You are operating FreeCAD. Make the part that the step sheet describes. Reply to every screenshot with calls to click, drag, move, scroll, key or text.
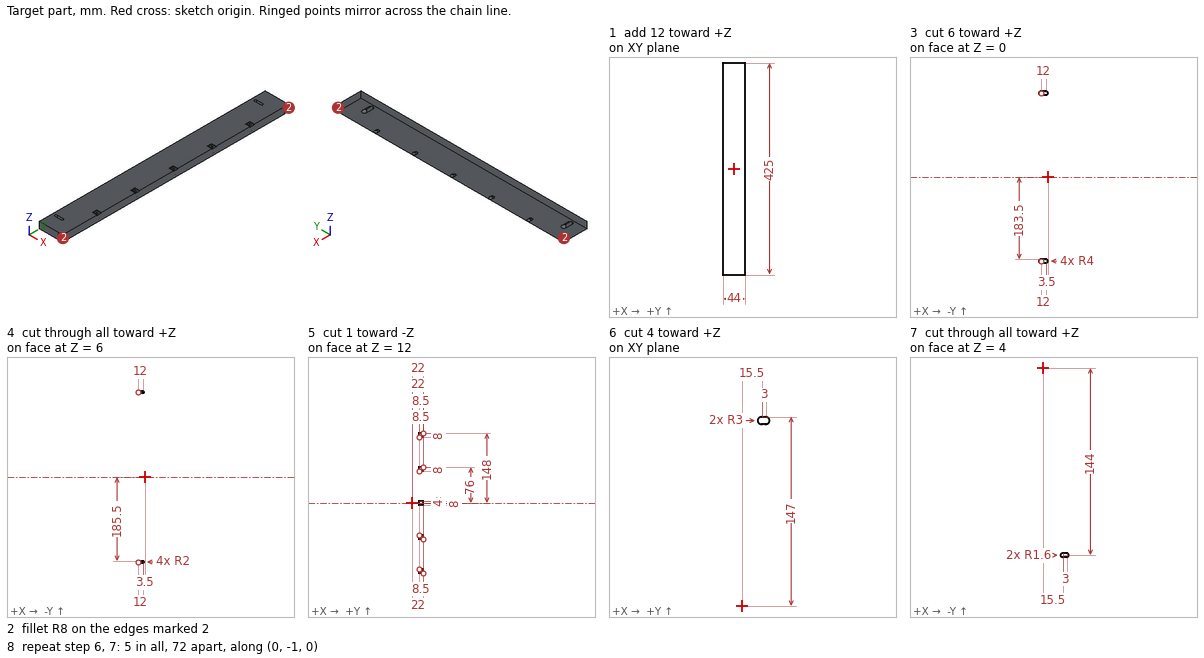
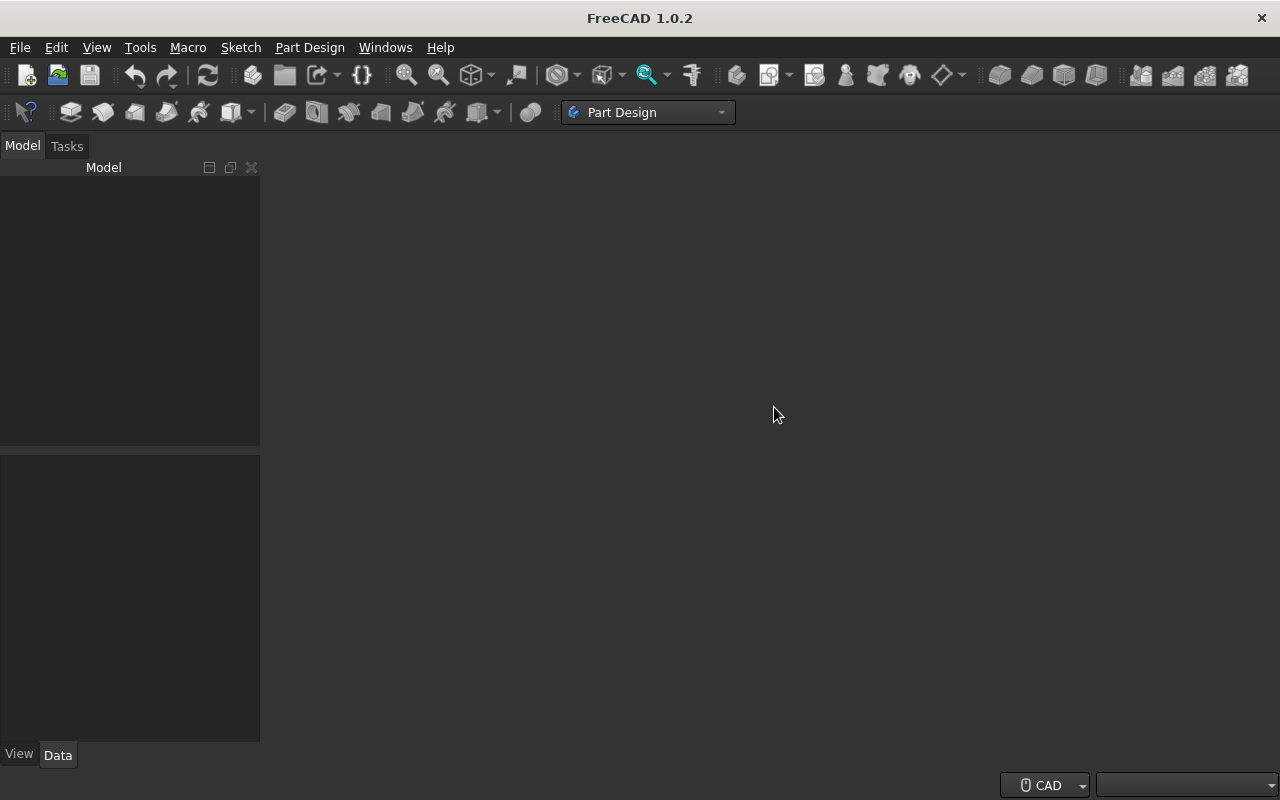
click(26, 76)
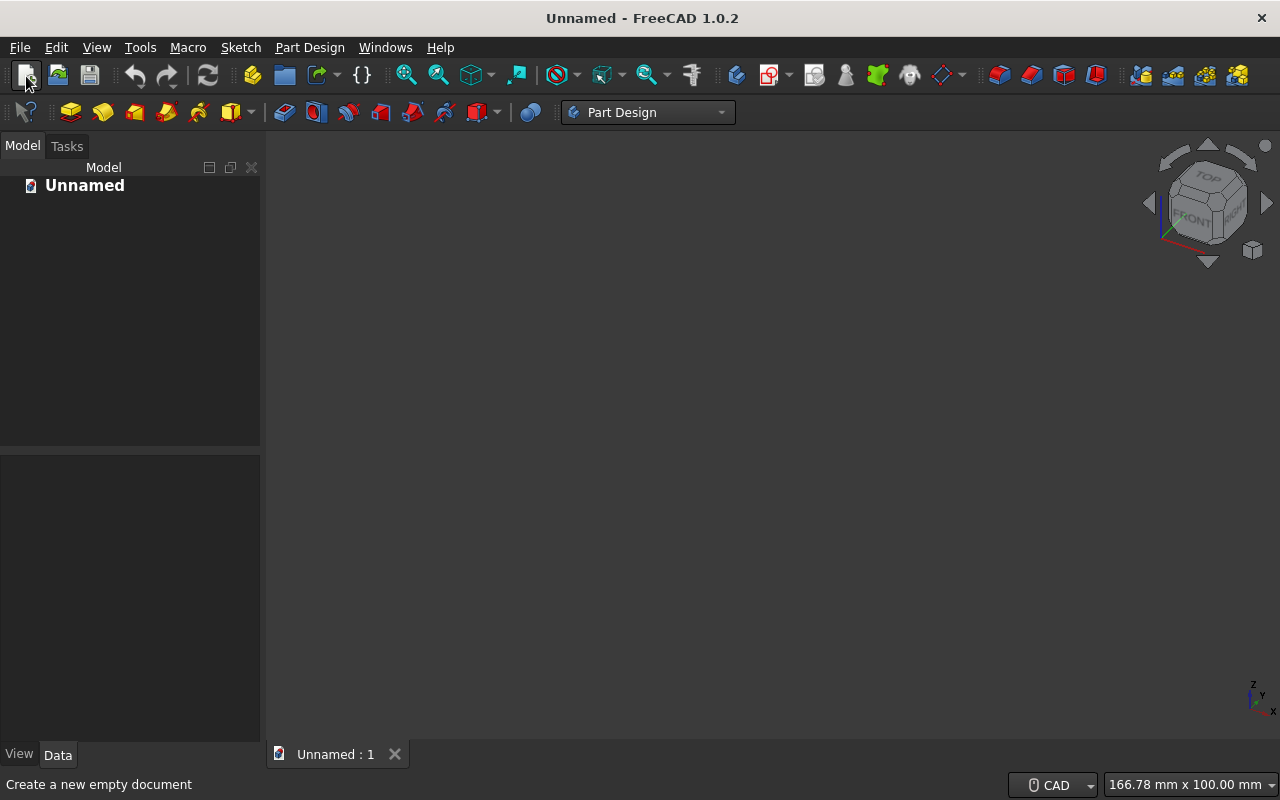
click(770, 76)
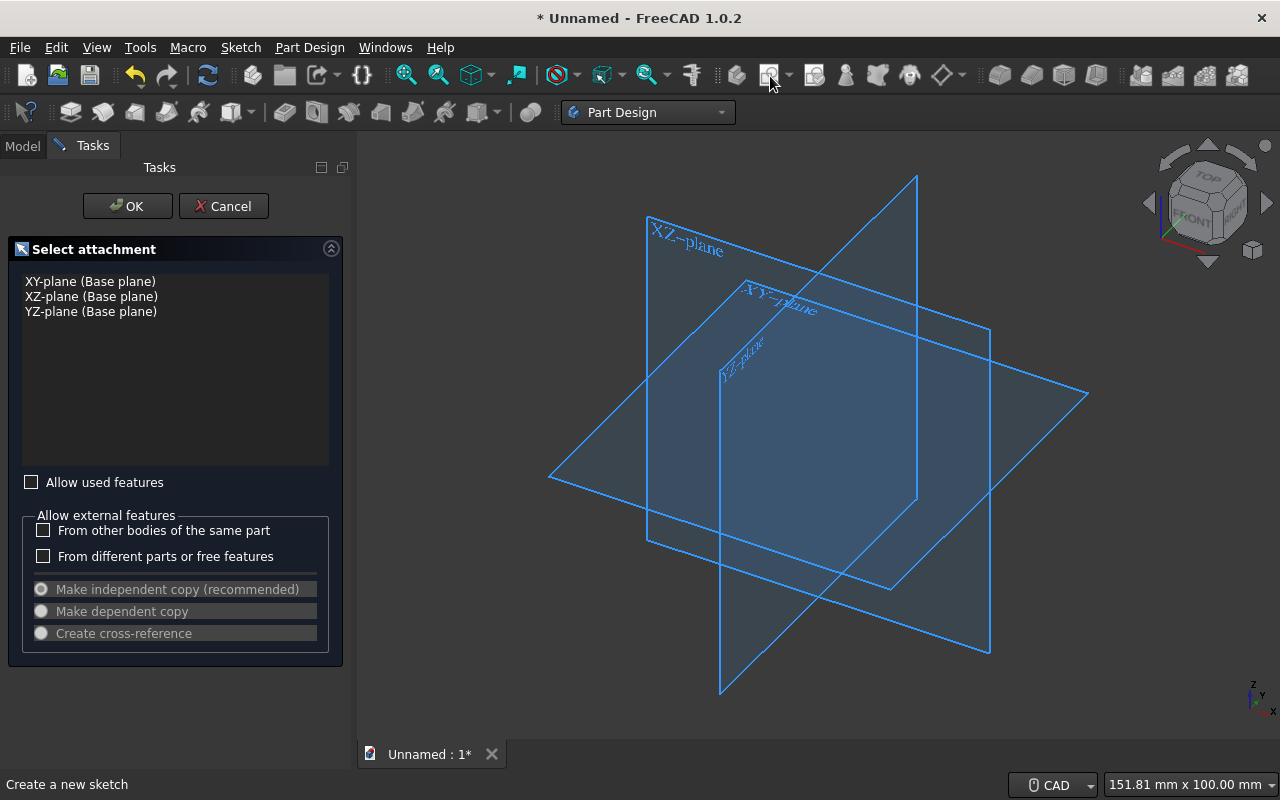
click(82, 282)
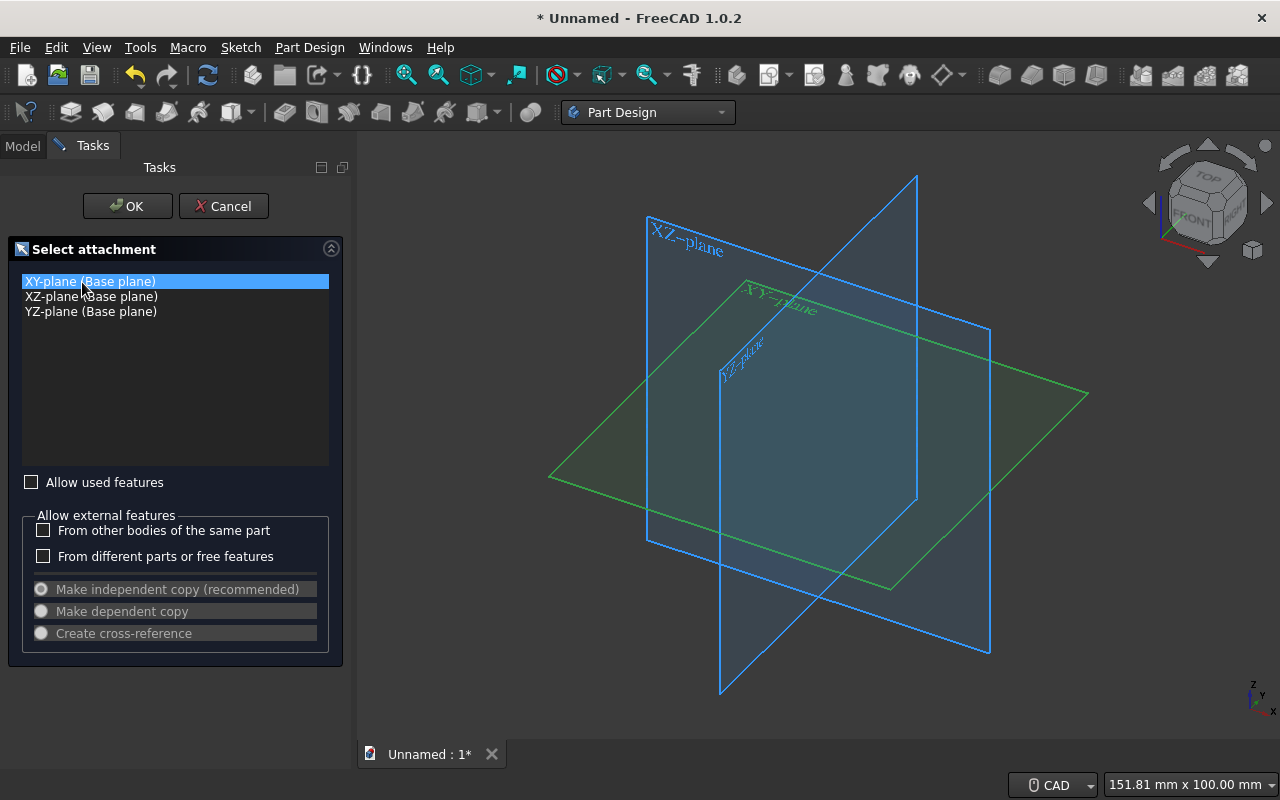
click(128, 206)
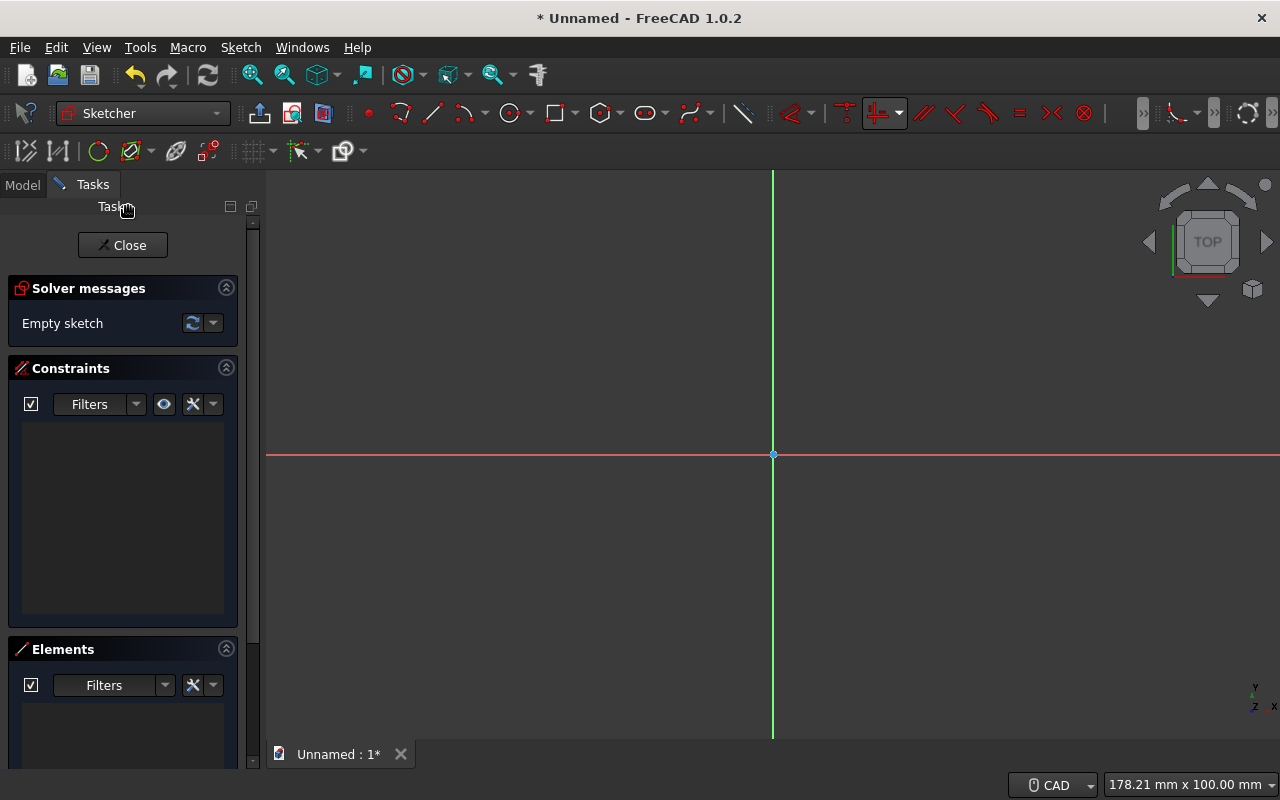
scroll(691, 454, down, 9)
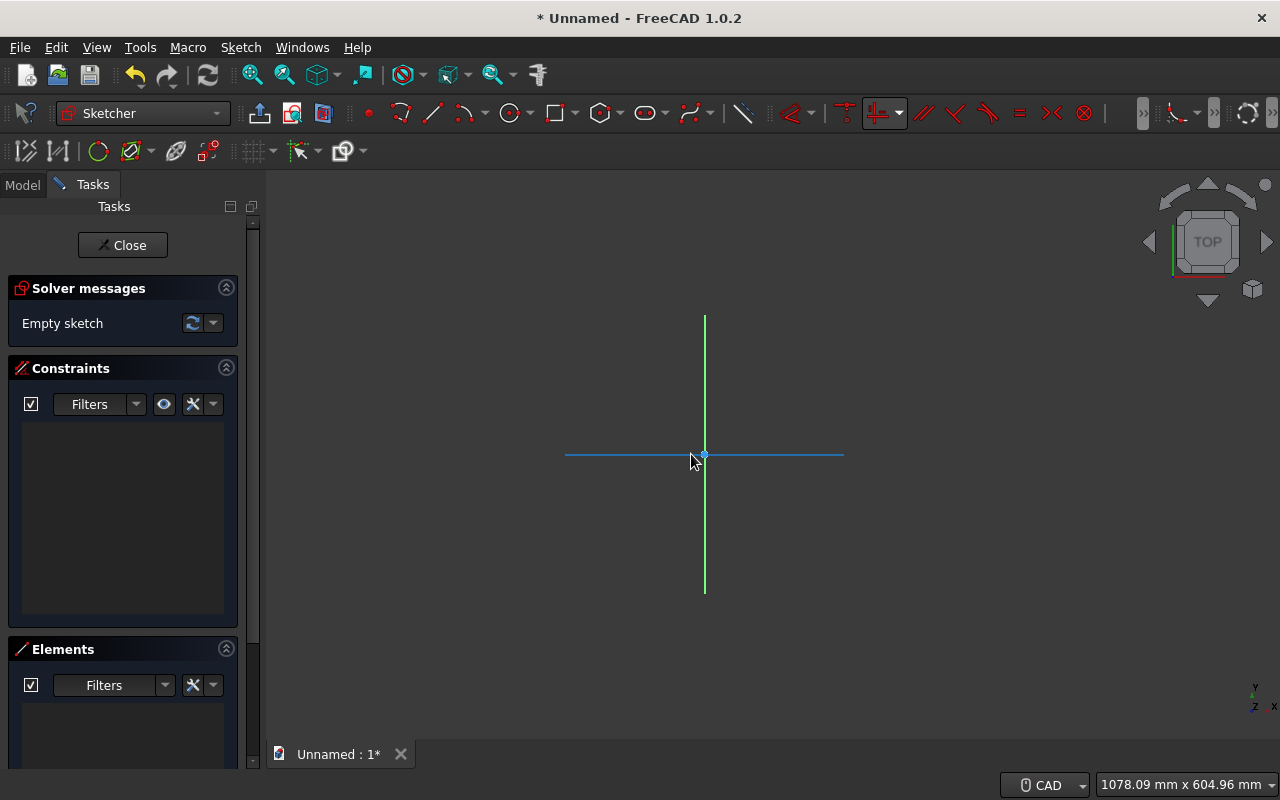
click(578, 114)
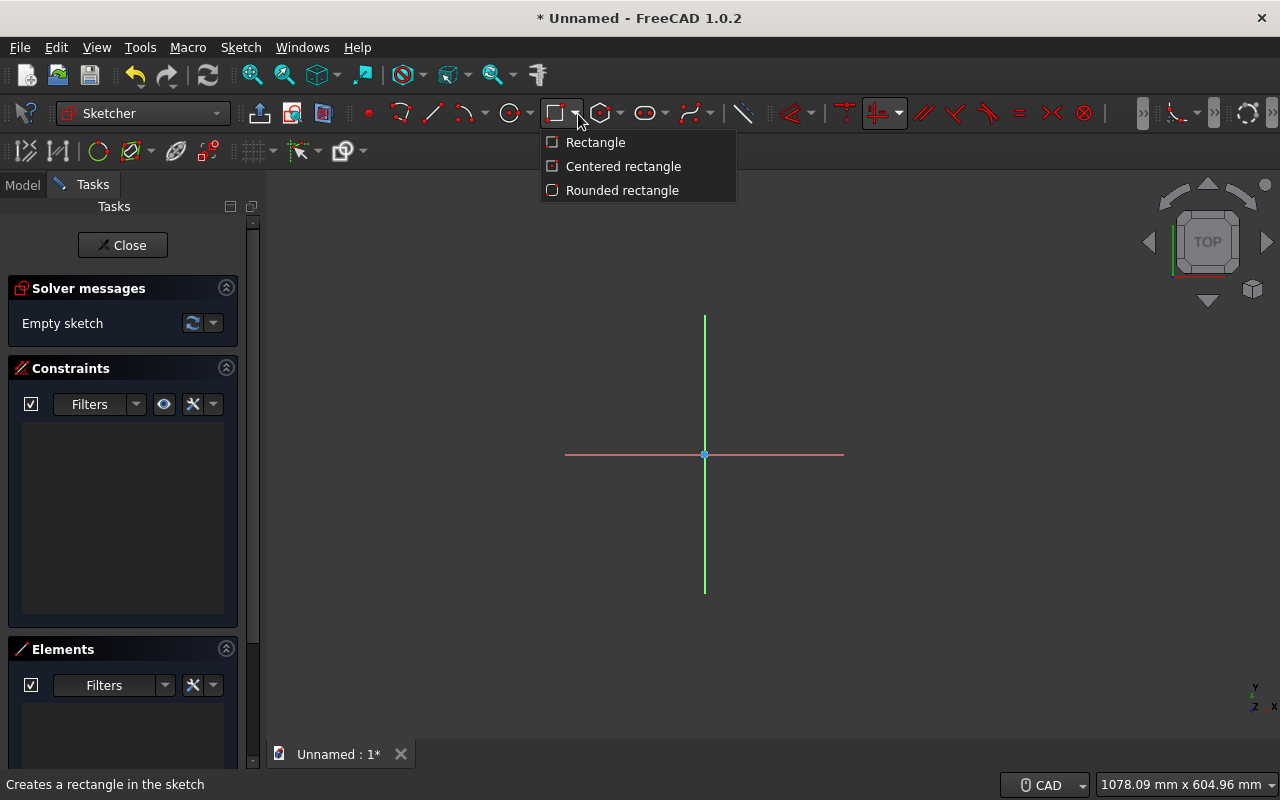
click(638, 166)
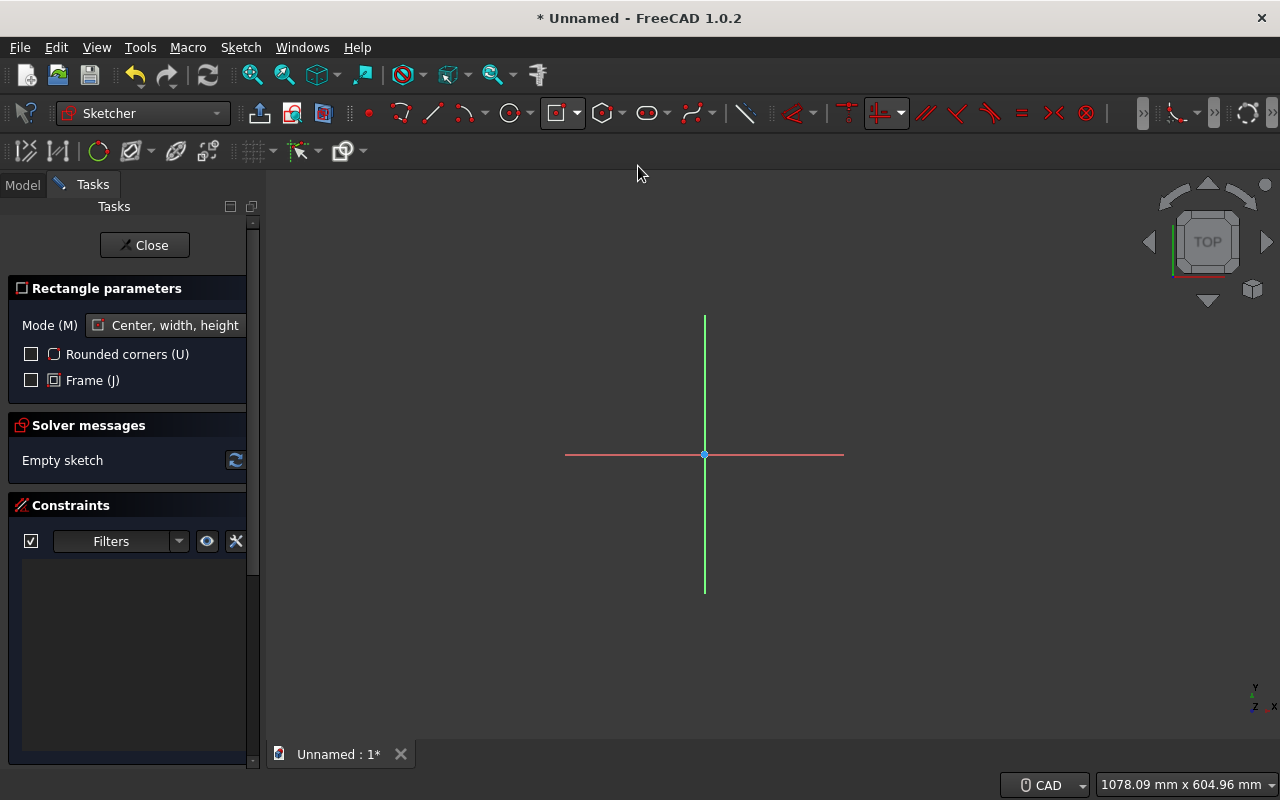
click(705, 454)
click(726, 255)
key(Escape)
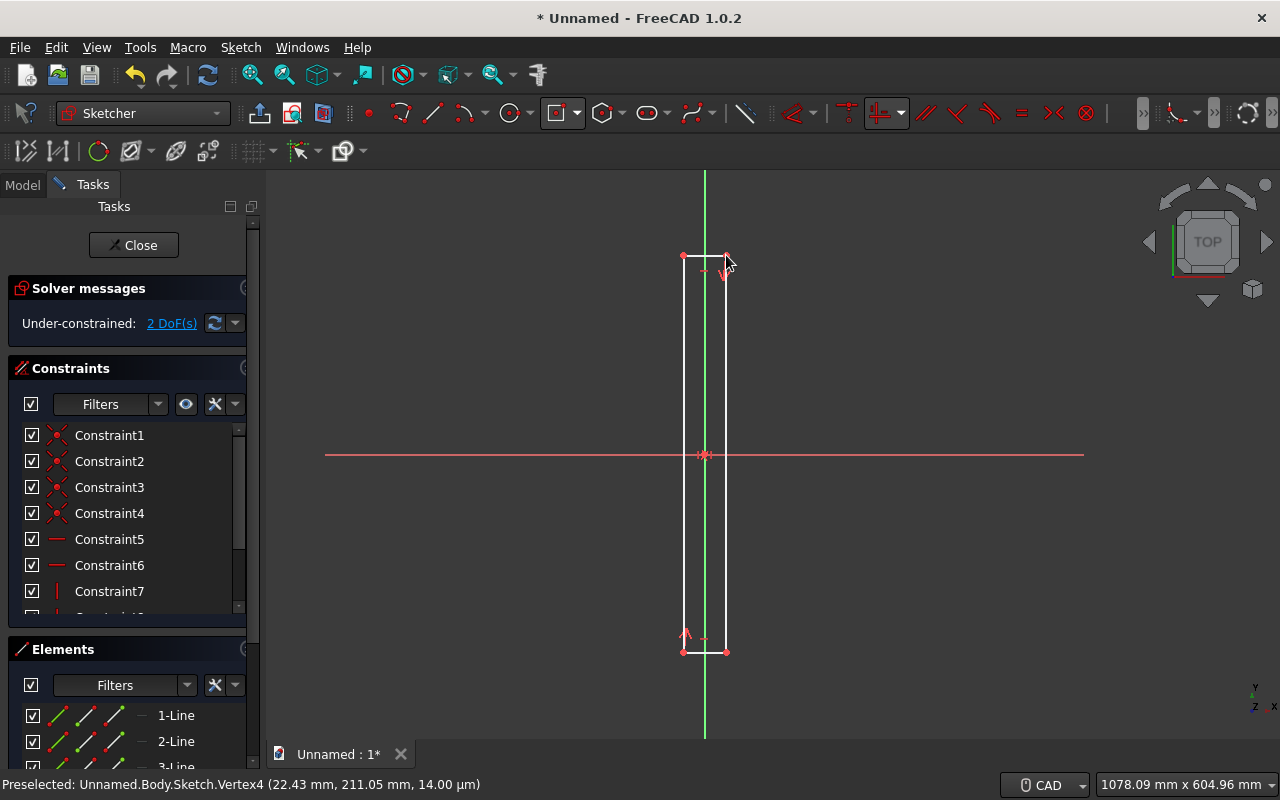
click(792, 114)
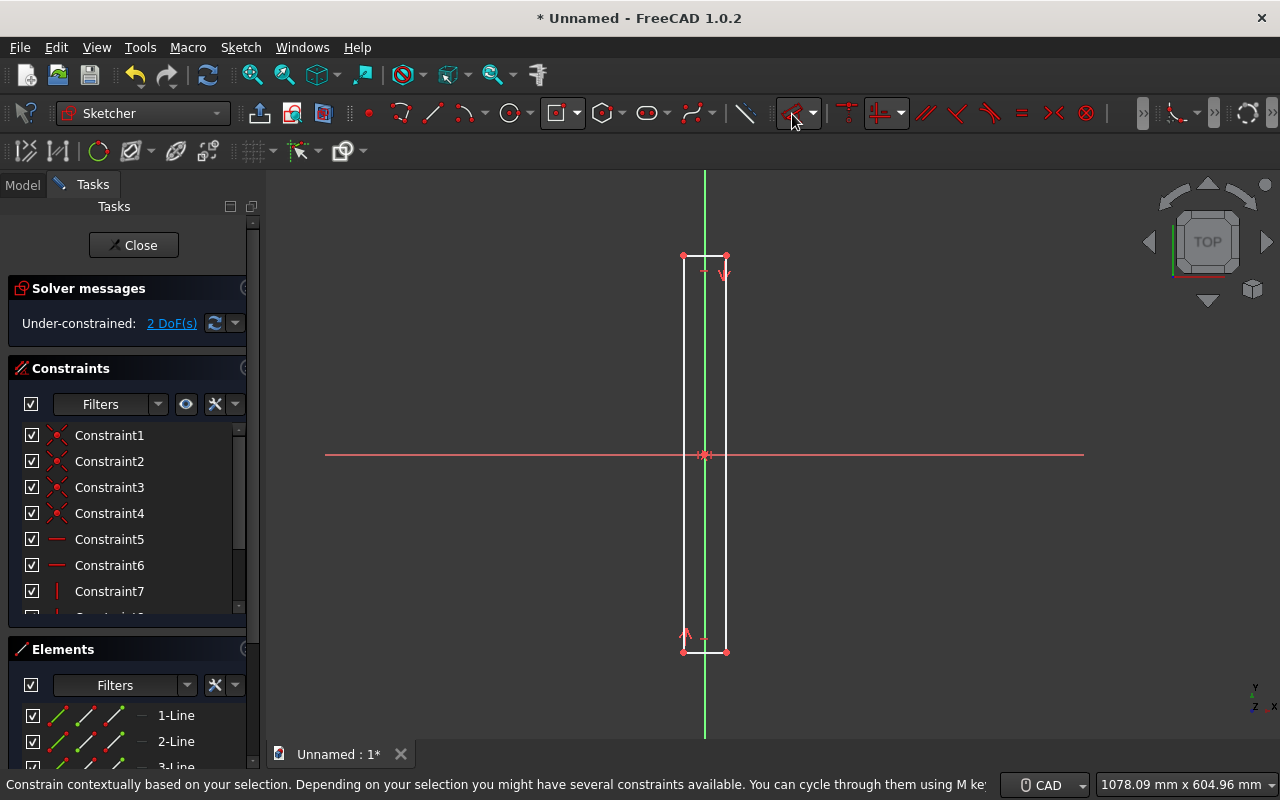
click(705, 653)
click(690, 687)